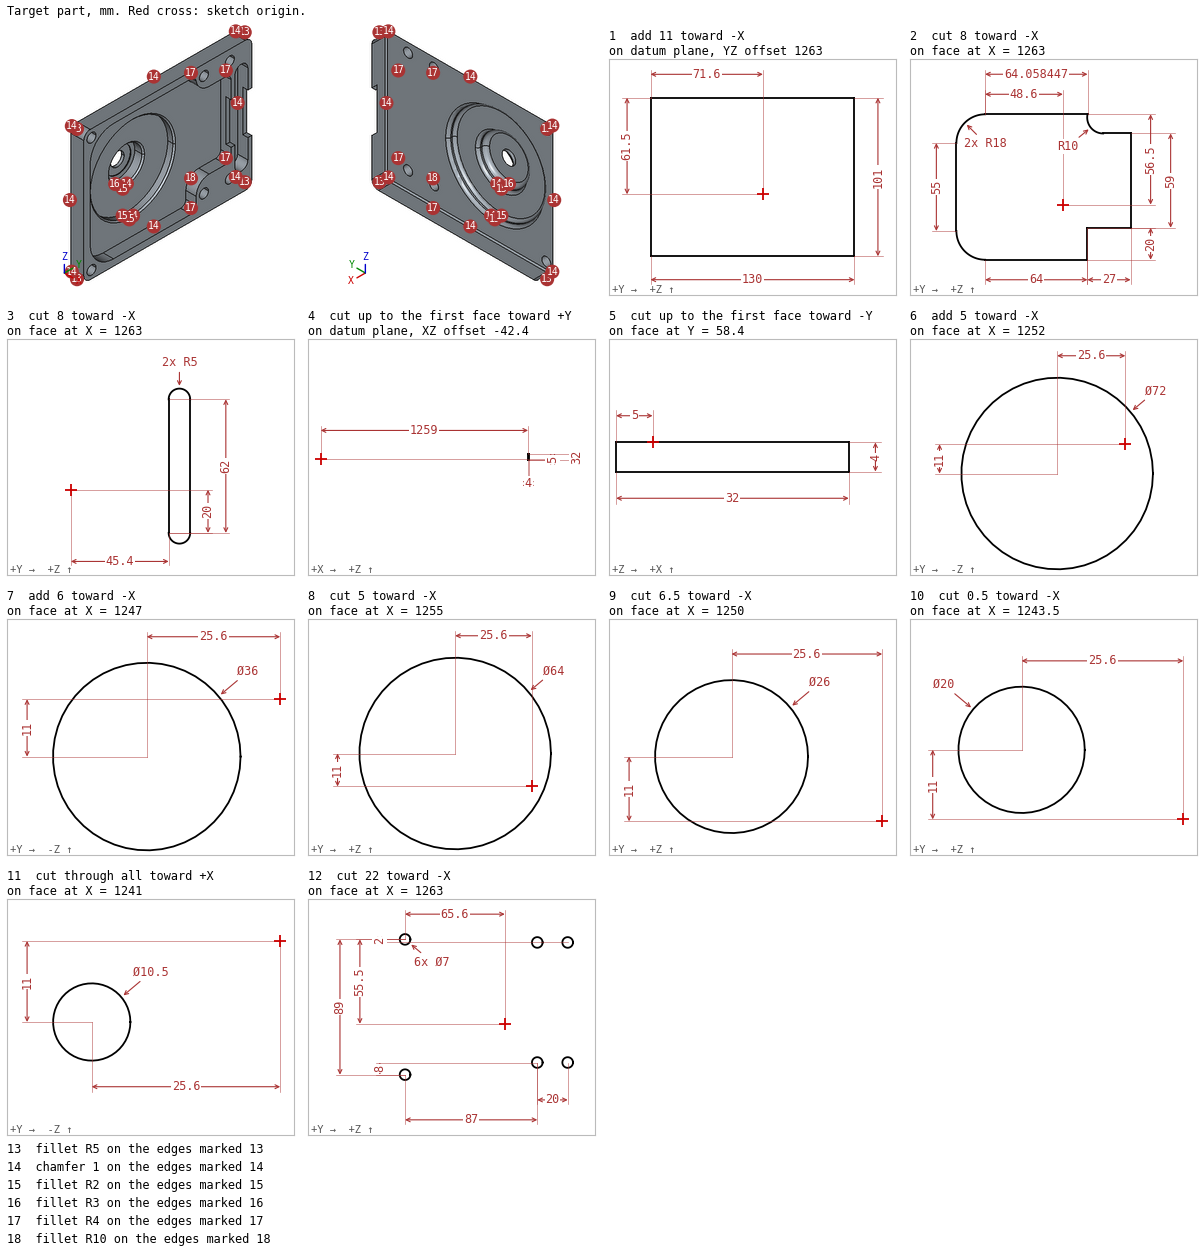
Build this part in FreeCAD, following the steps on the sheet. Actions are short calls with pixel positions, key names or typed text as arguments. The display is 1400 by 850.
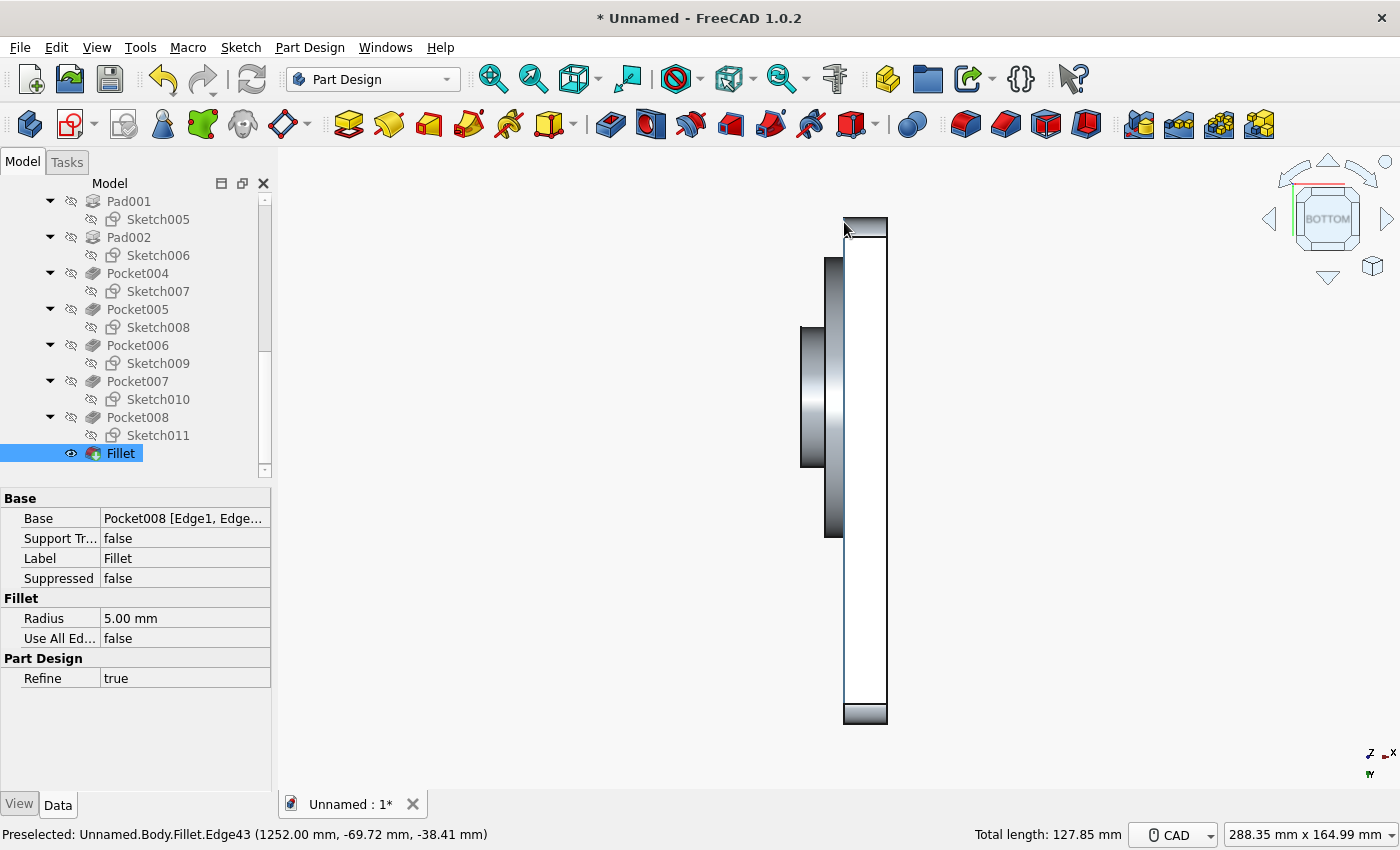
click(844, 717, ctrl)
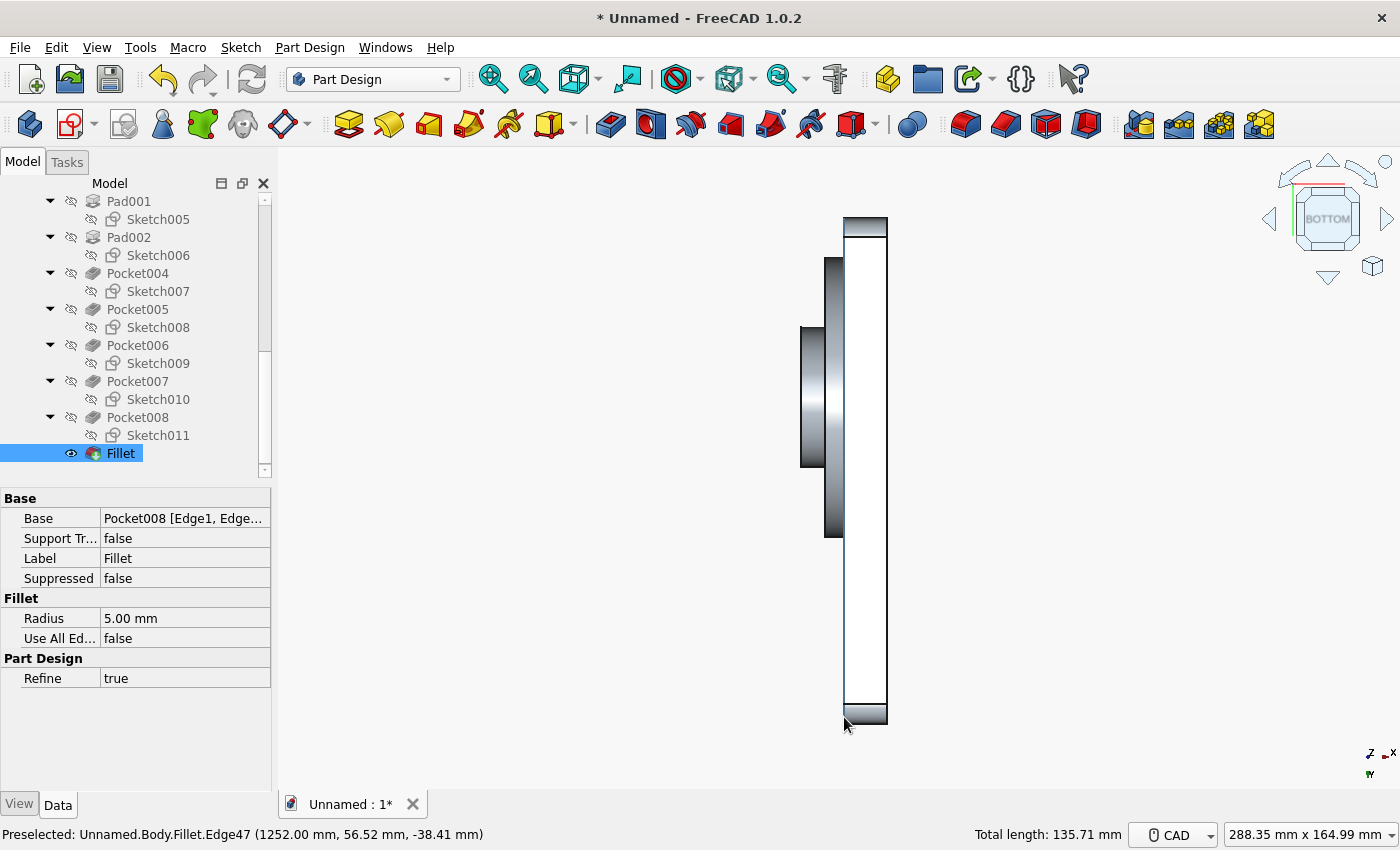
key(0)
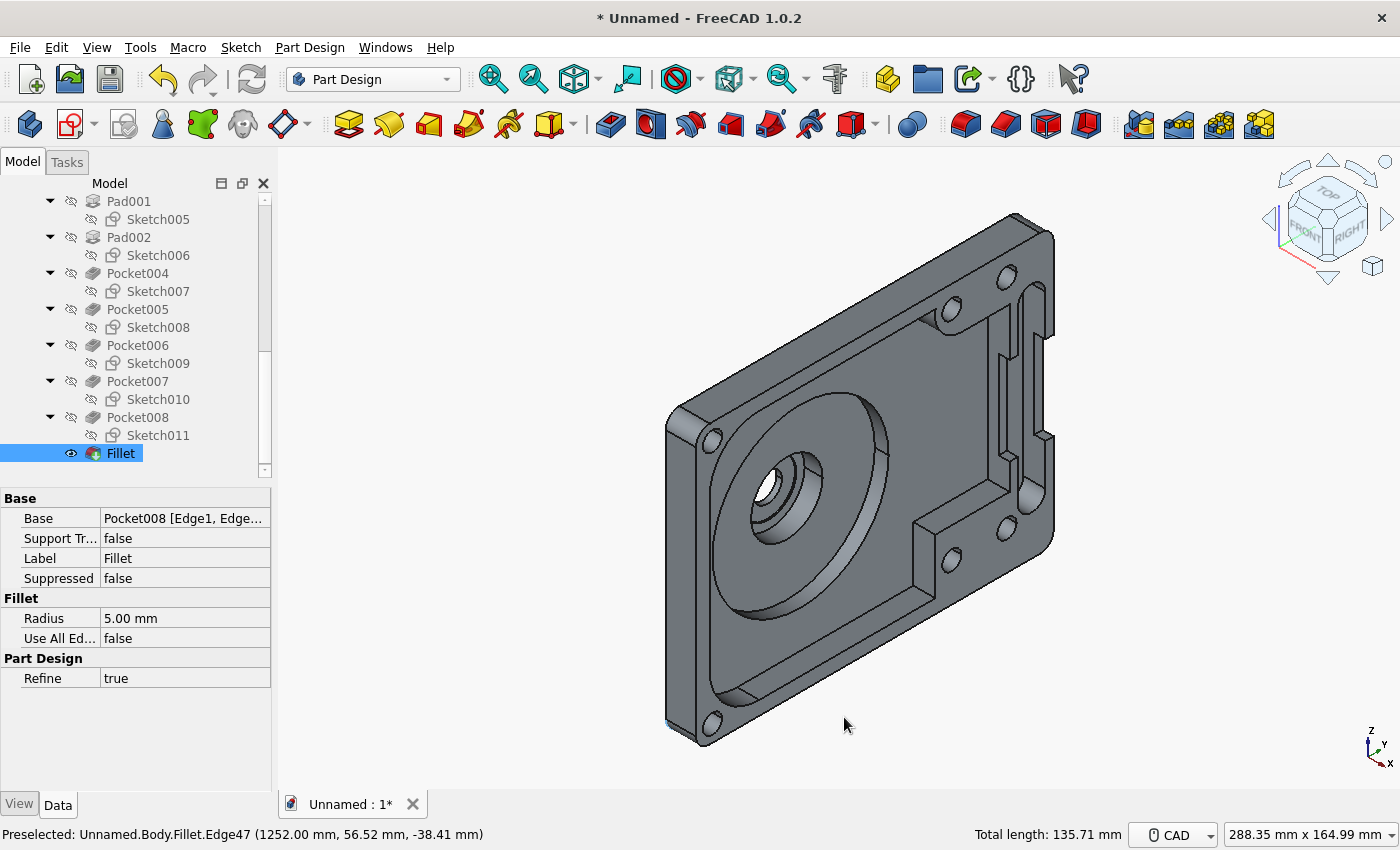
click(667, 421, ctrl)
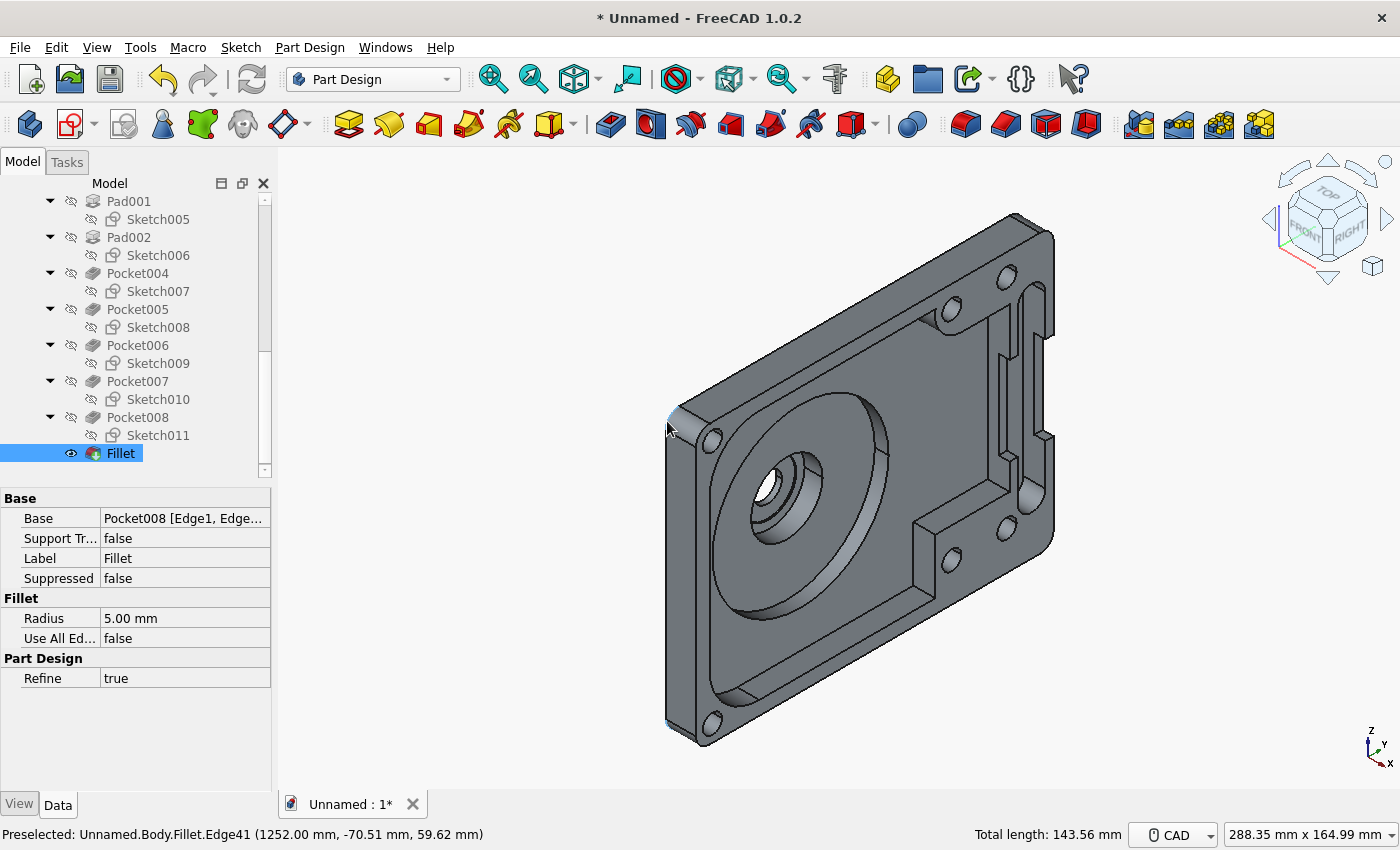
click(773, 618, ctrl)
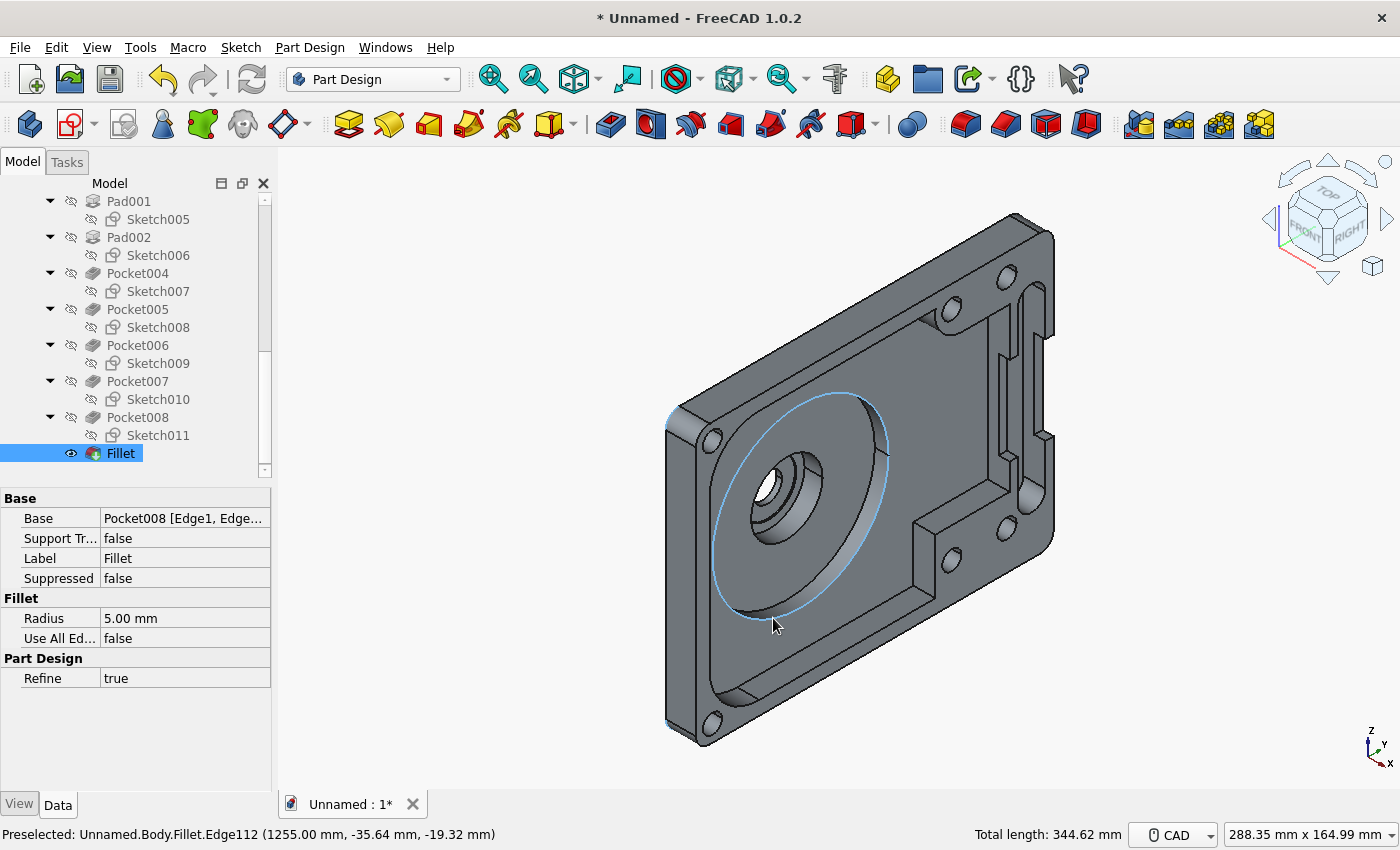
click(776, 543, ctrl)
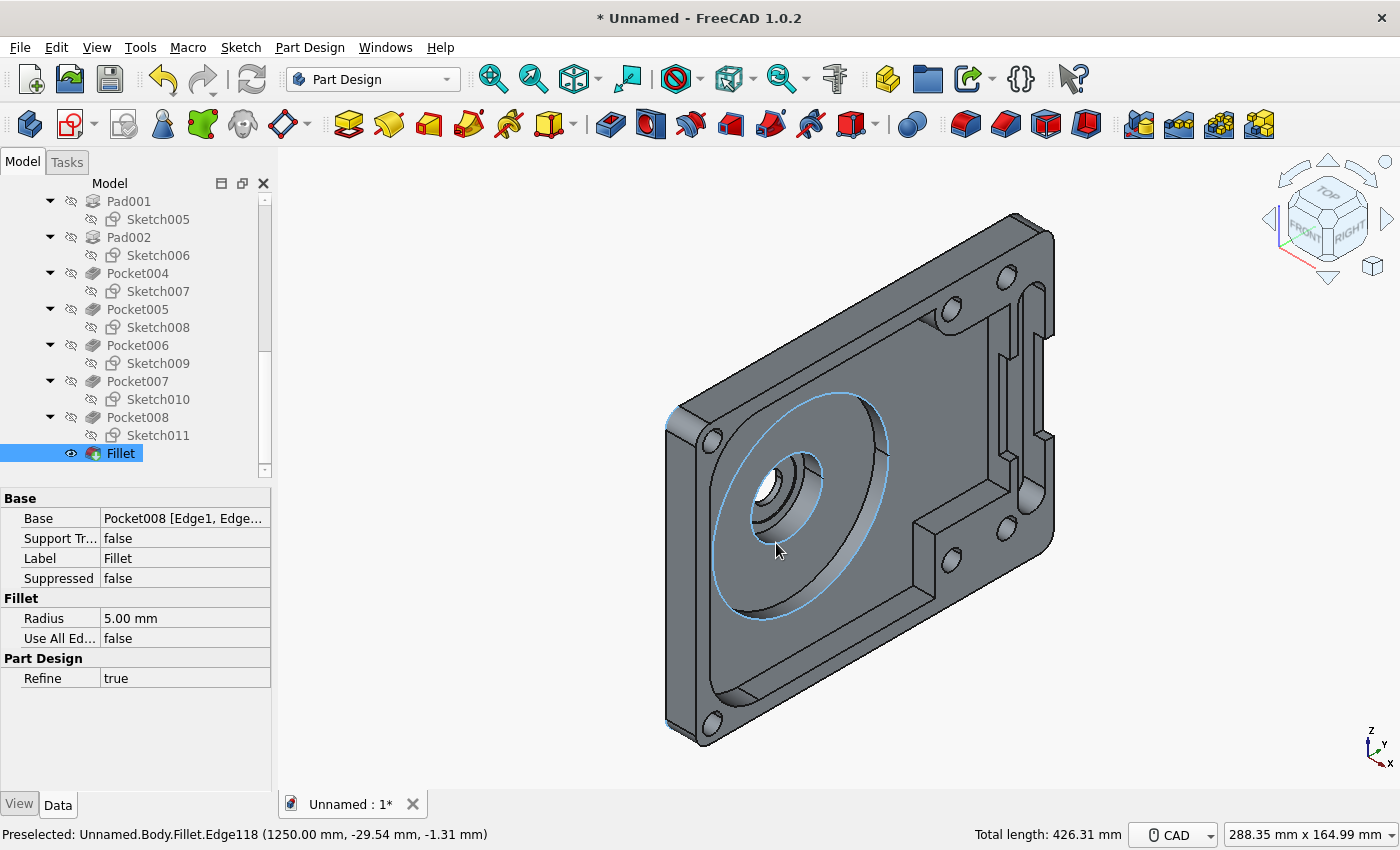
key(2)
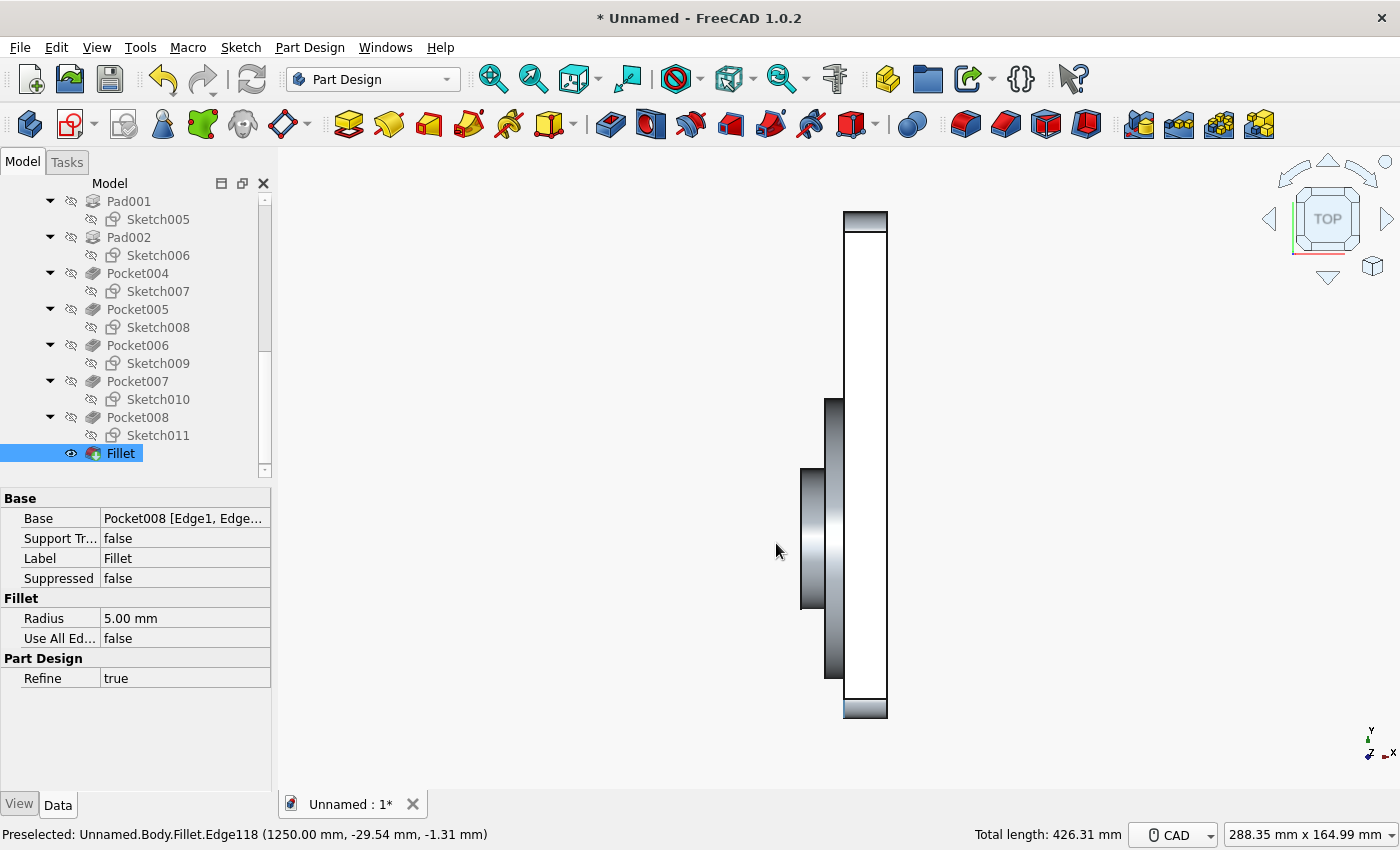
click(844, 464, ctrl)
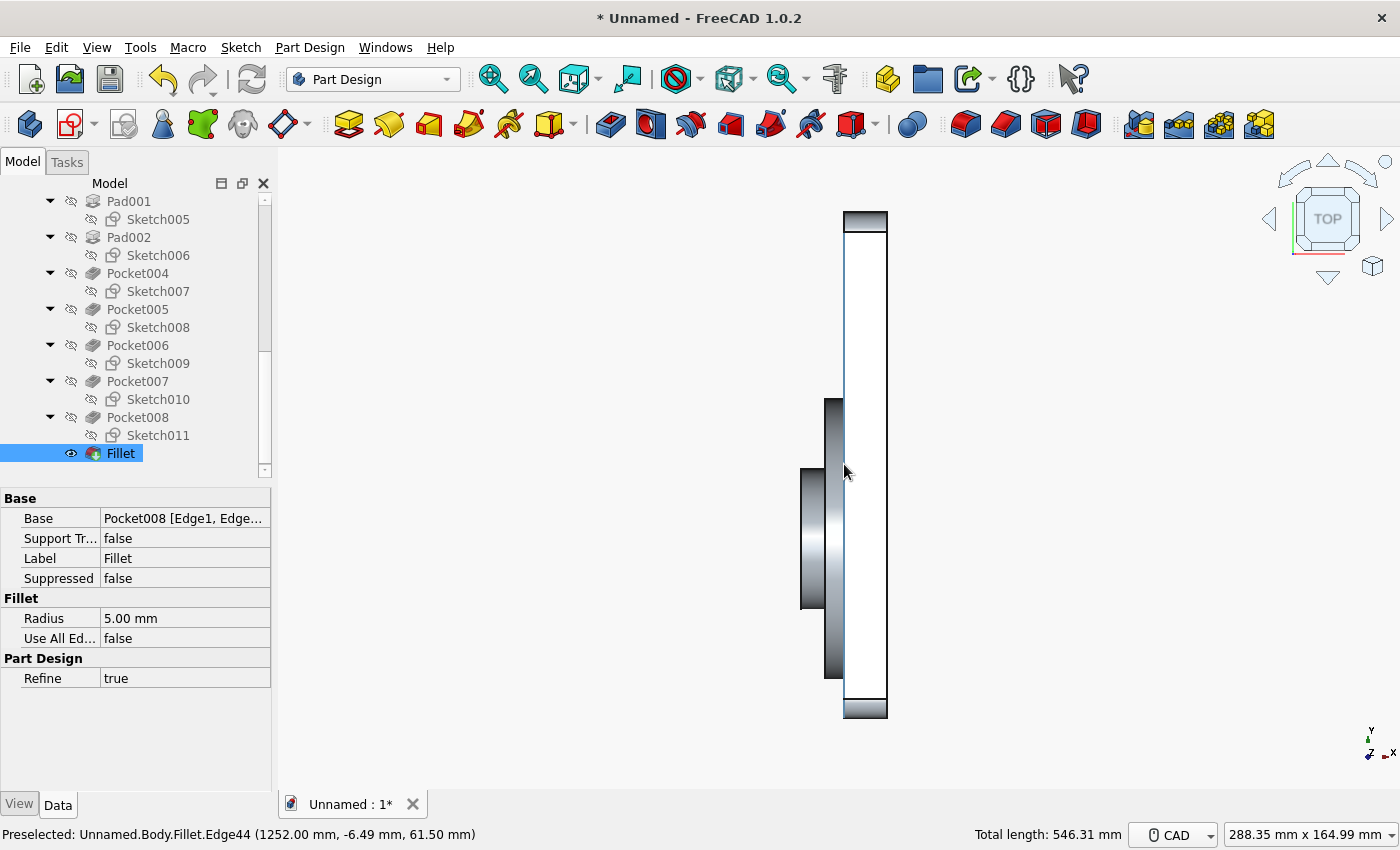
click(844, 217, ctrl)